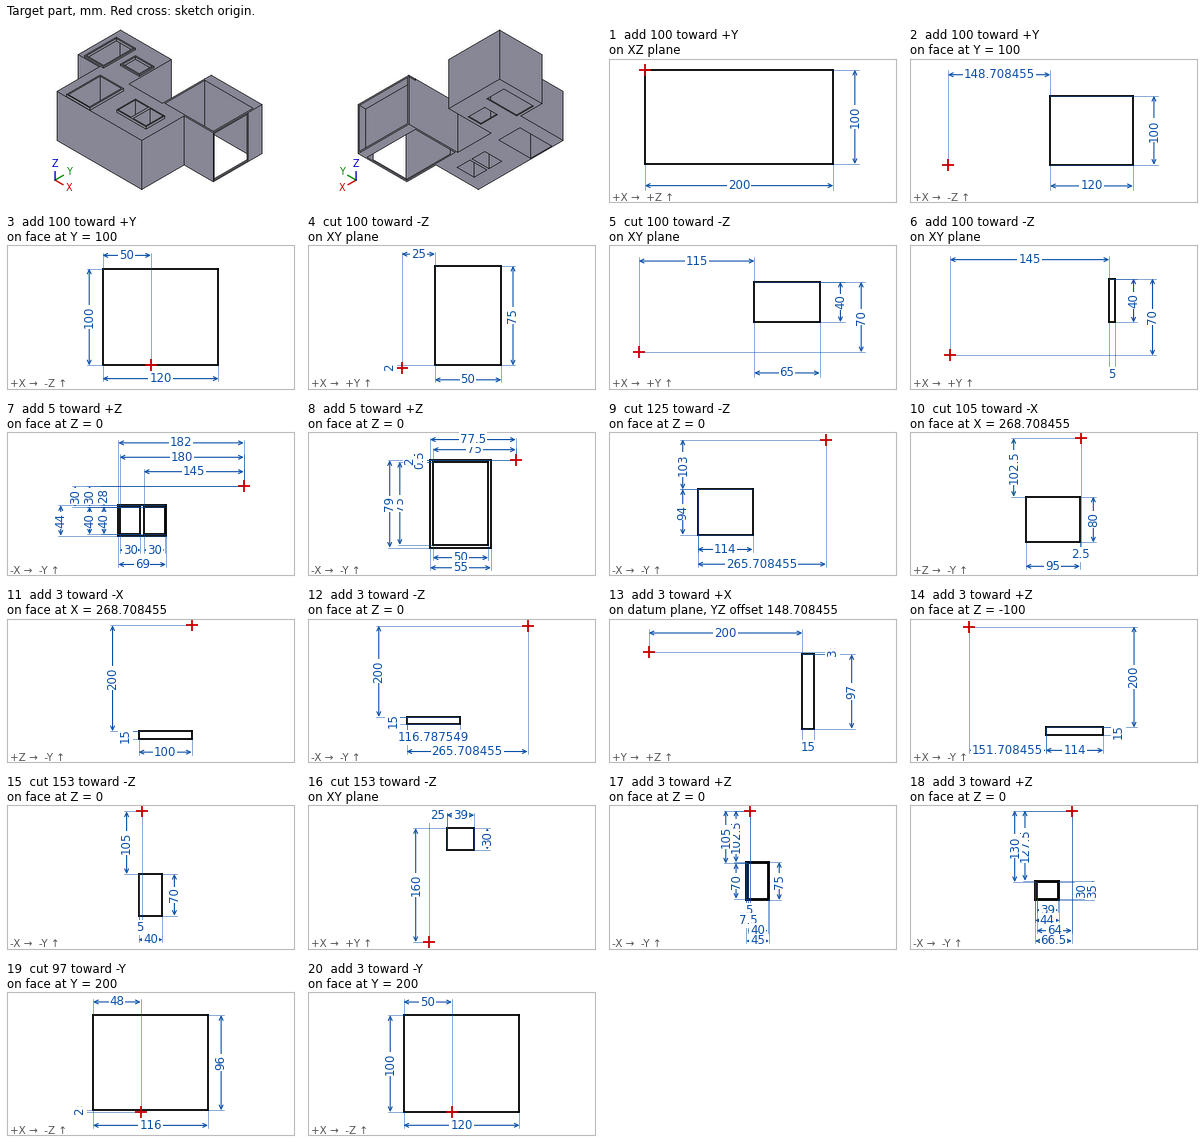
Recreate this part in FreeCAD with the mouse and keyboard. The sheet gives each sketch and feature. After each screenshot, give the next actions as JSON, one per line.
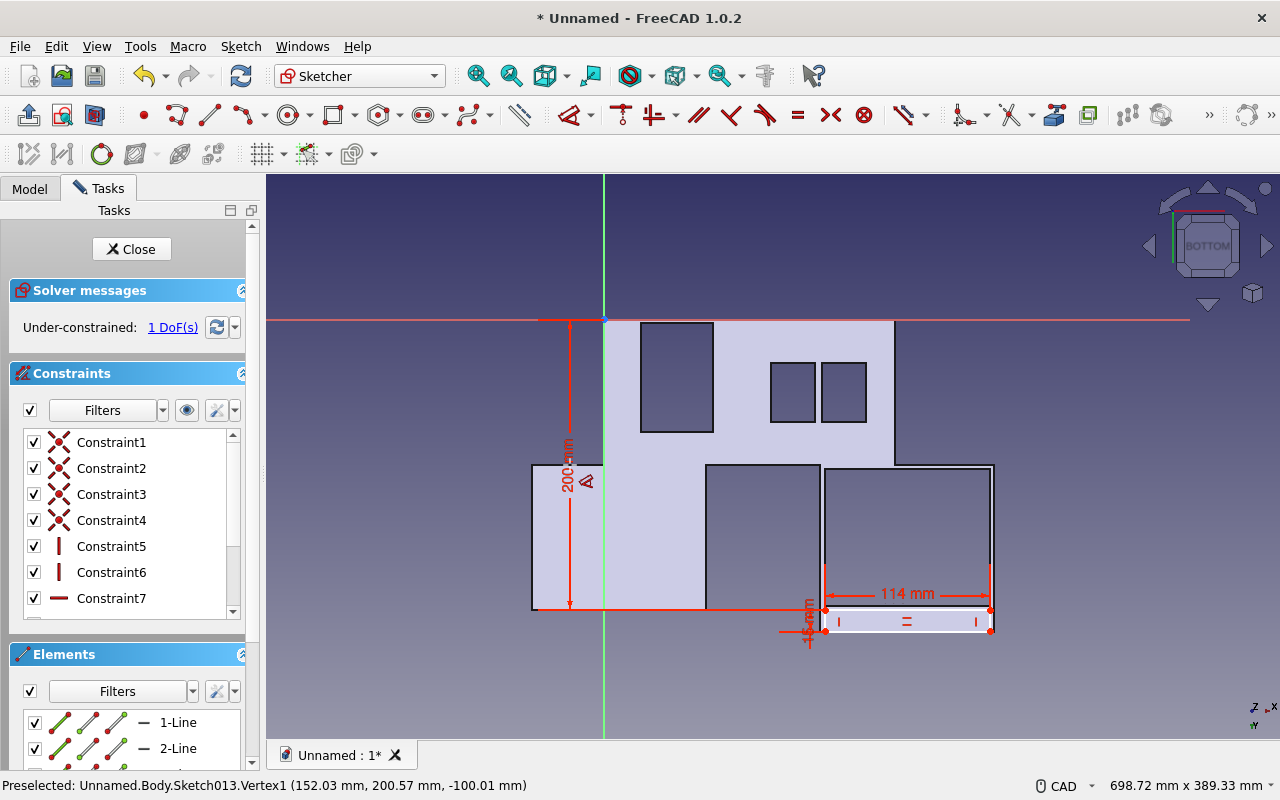
{"action": "left_click", "coordinate": [825, 610]}
{"action": "left_click", "coordinate": [715, 286]}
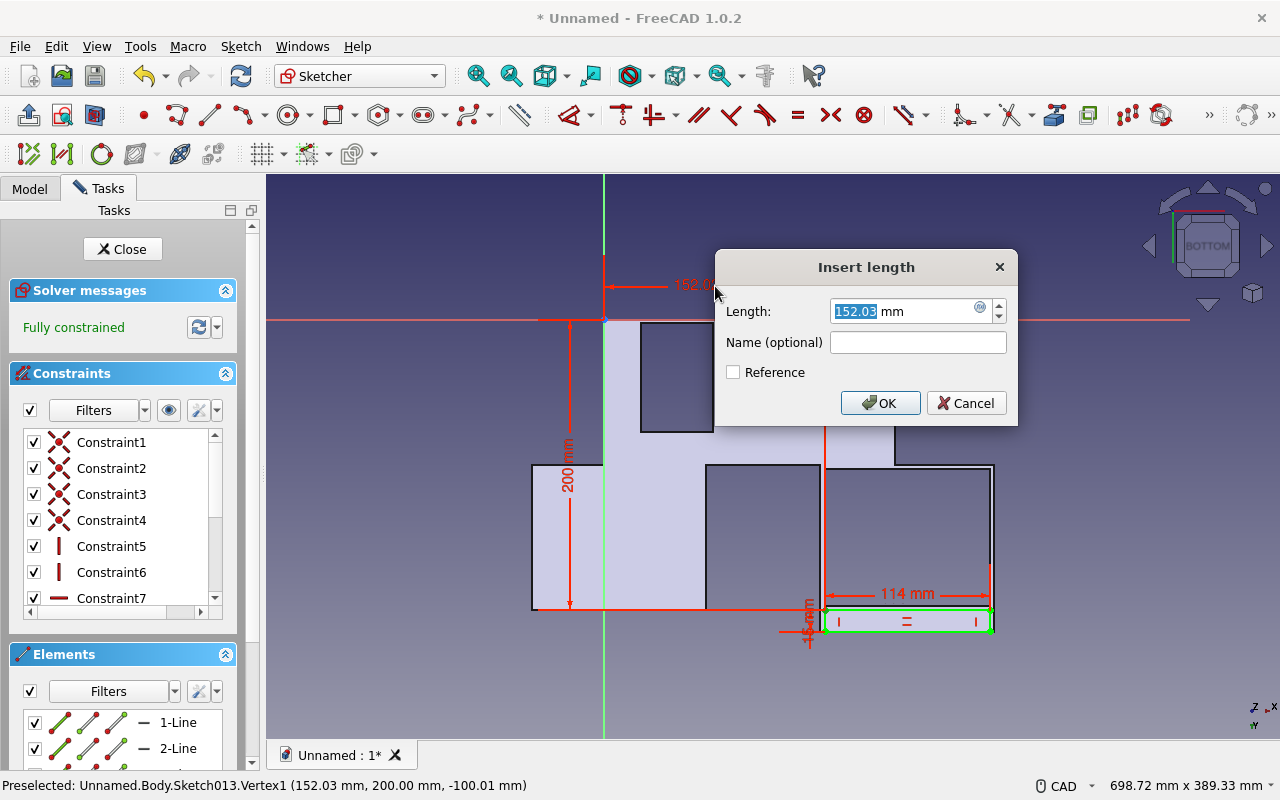
{"action": "type", "text": "151.708455"}
{"action": "key", "text": "Return"}
{"action": "key", "text": "Escape"}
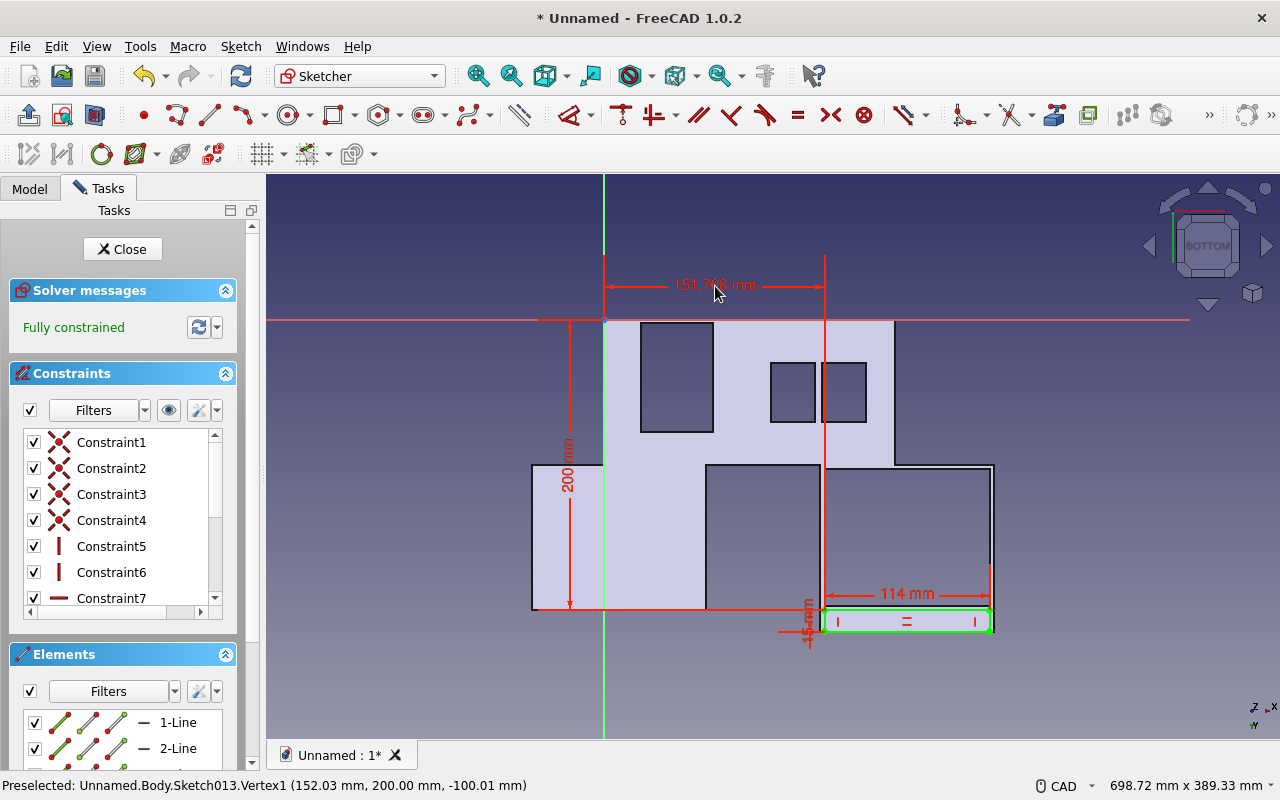
{"action": "left_click", "coordinate": [123, 249]}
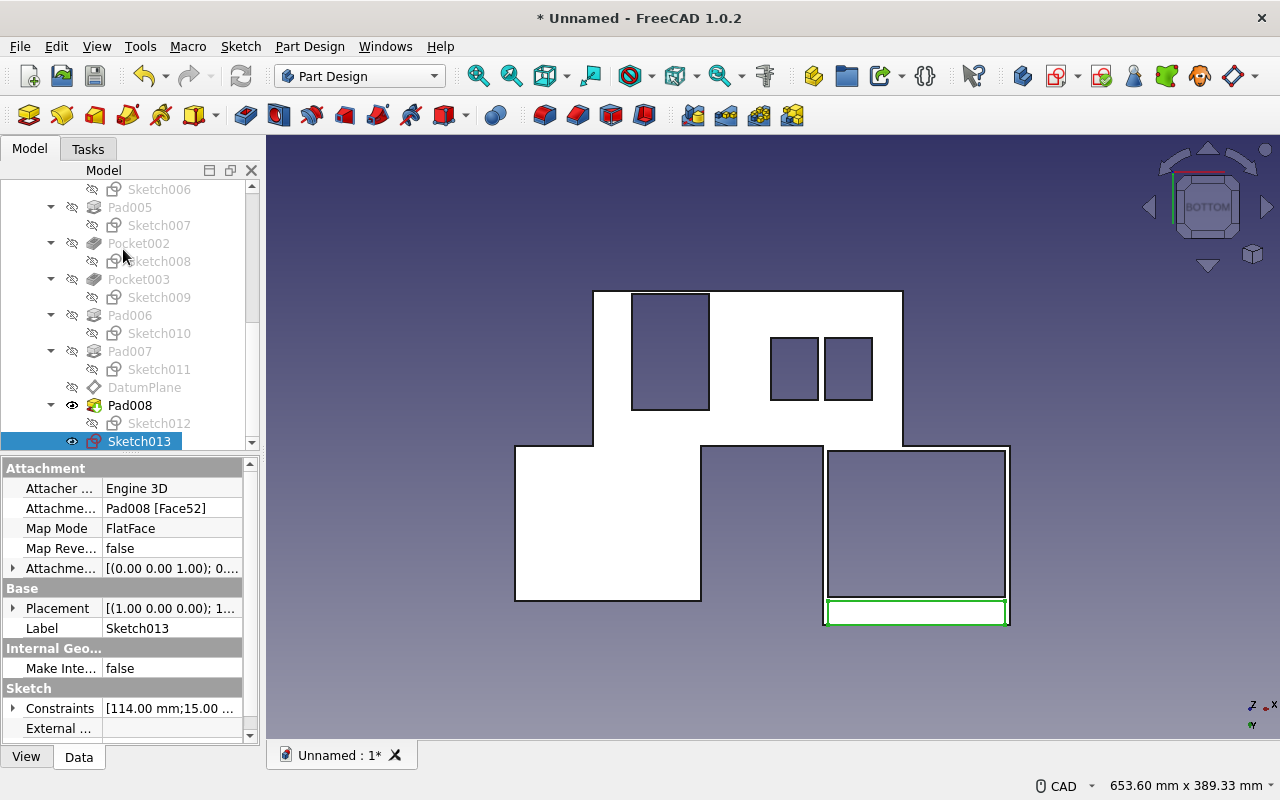
{"action": "left_click", "coordinate": [29, 116]}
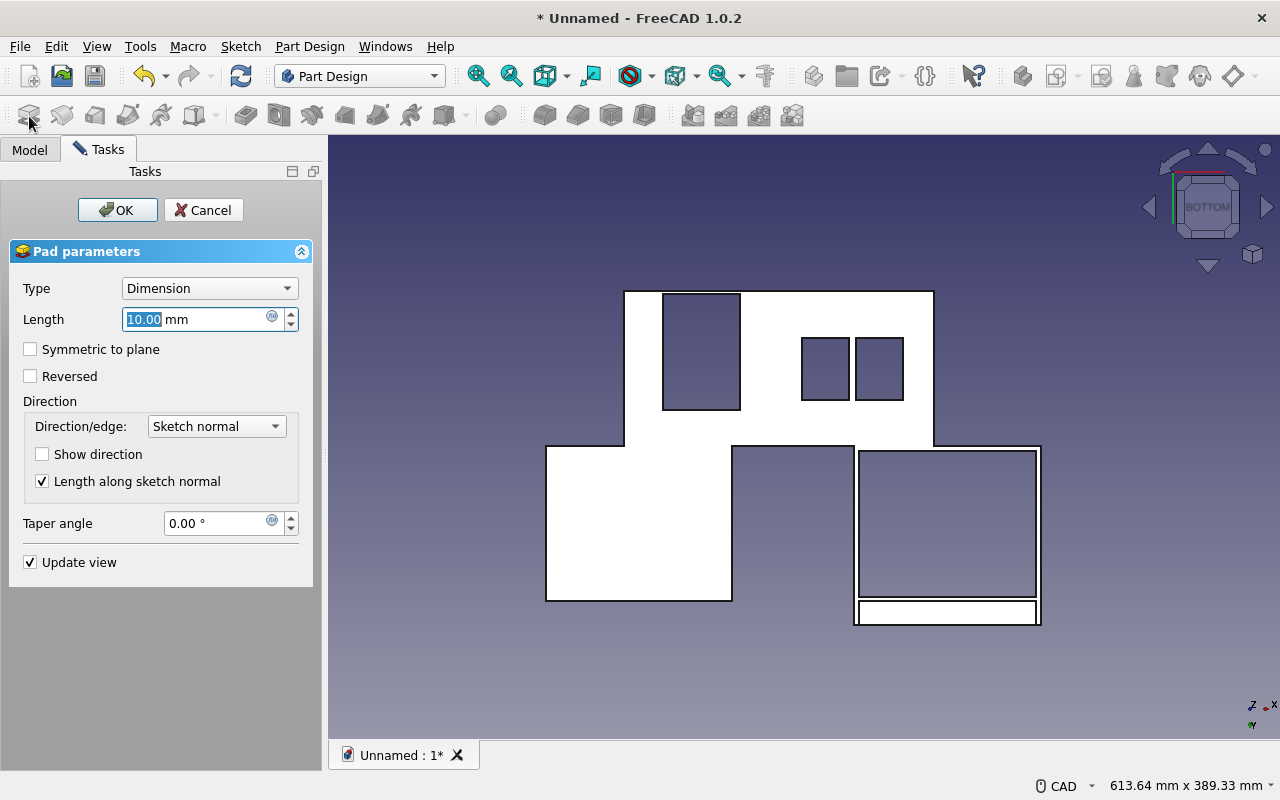
{"action": "type", "text": "3"}
{"action": "key", "text": "Tab"}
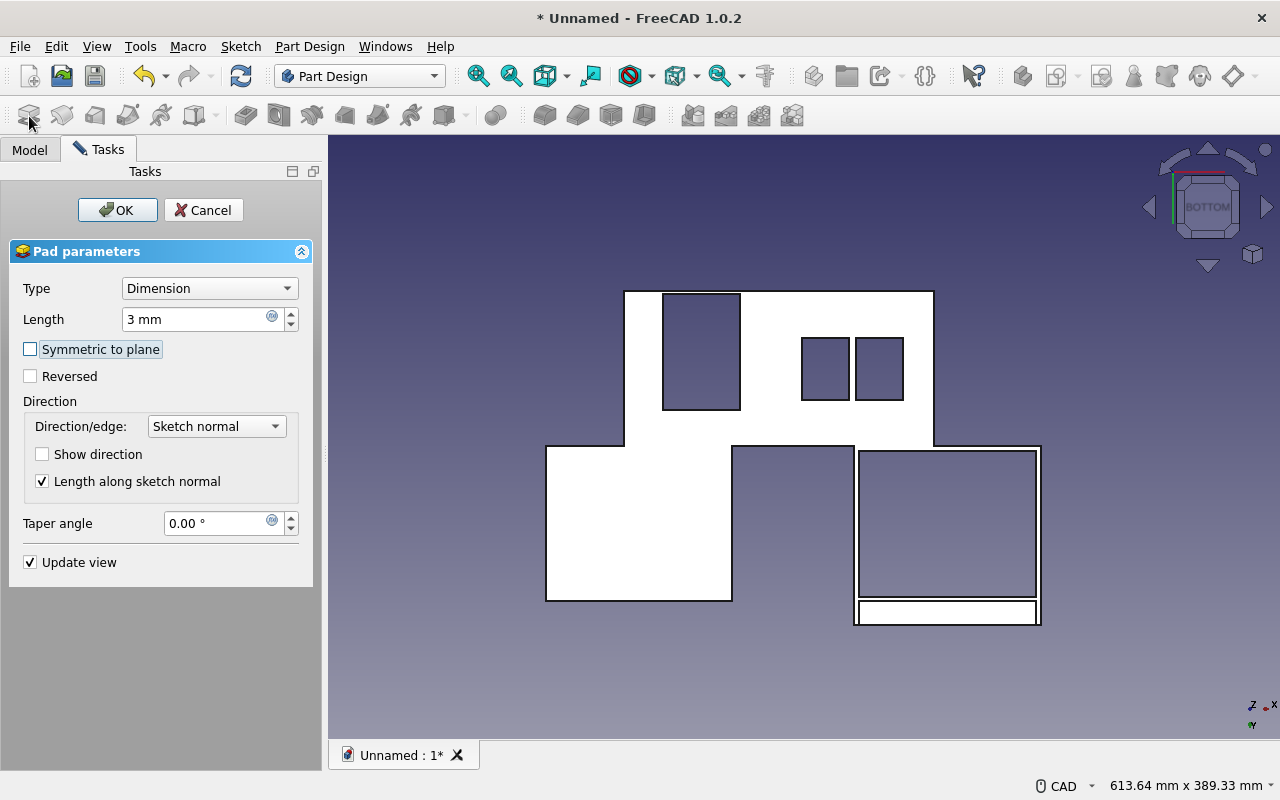
{"action": "left_click", "coordinate": [31, 376]}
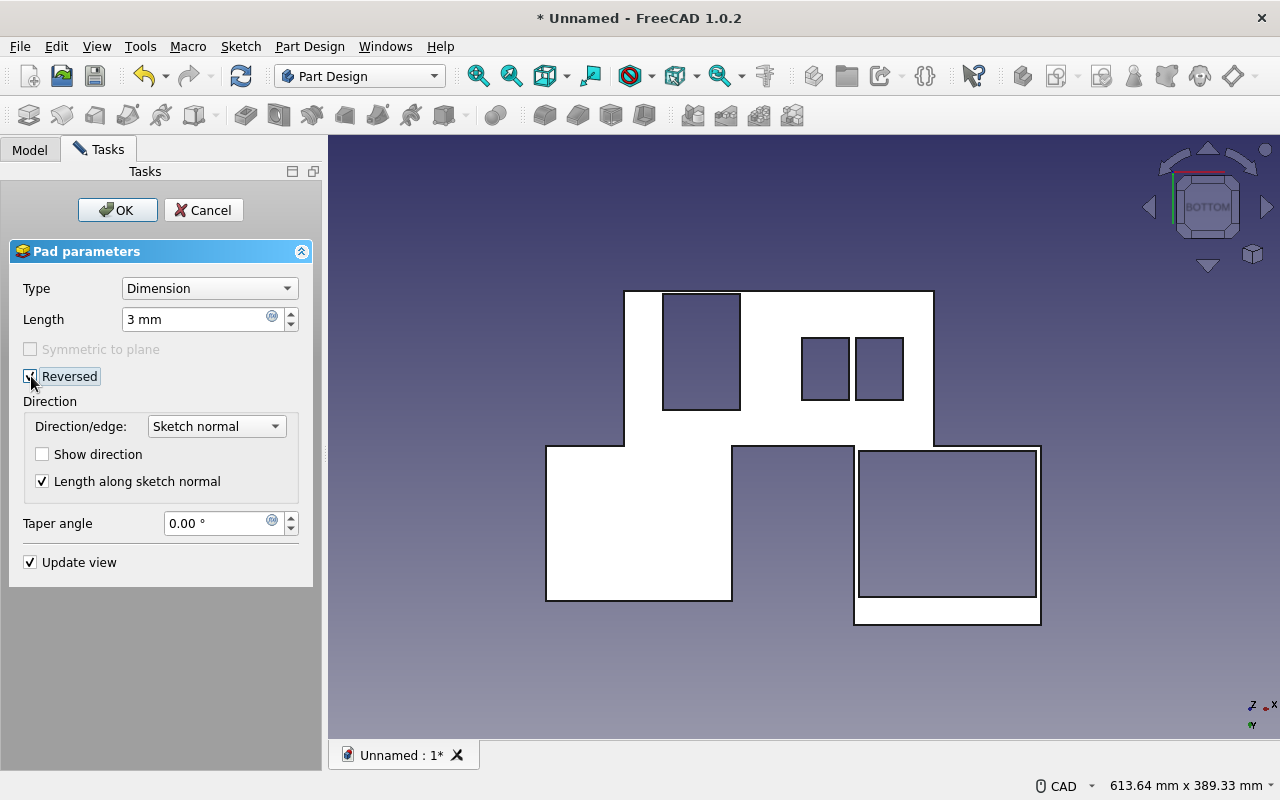
{"action": "left_click", "coordinate": [118, 210]}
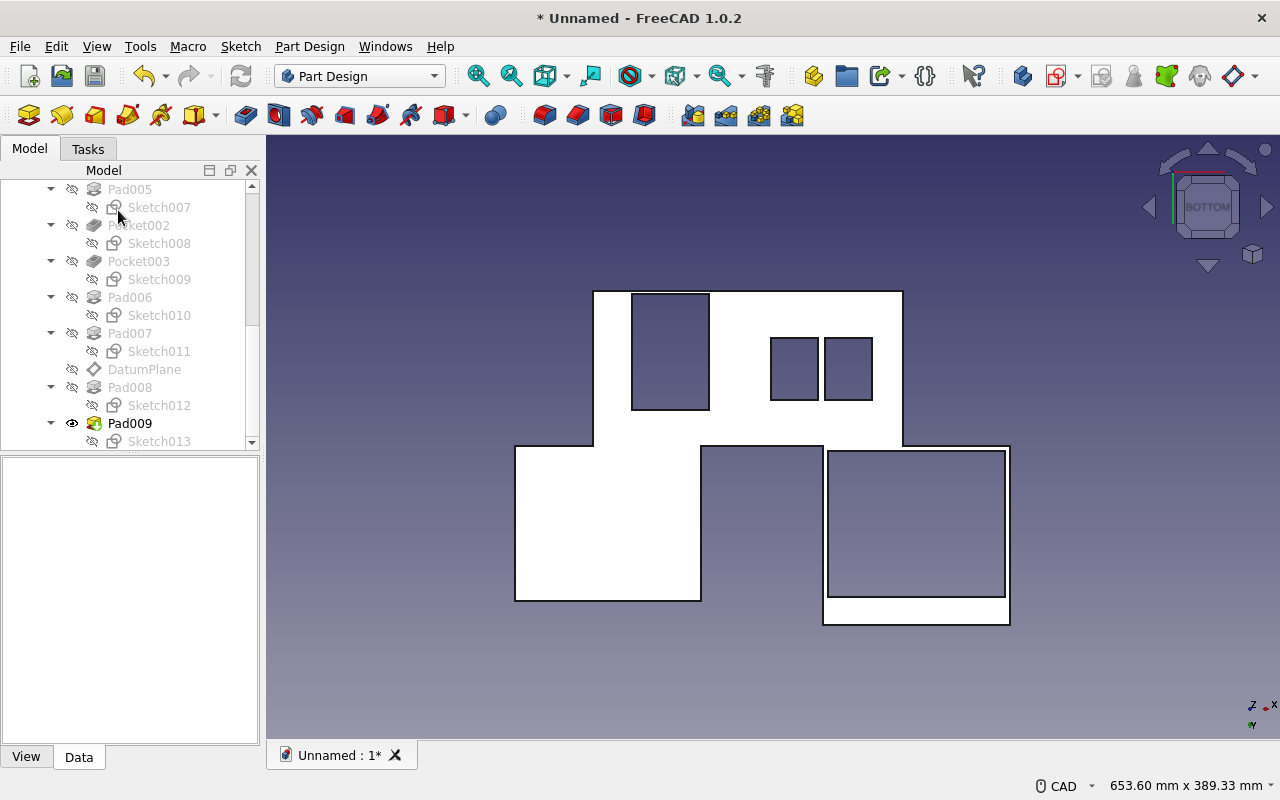
{"action": "key", "text": "0"}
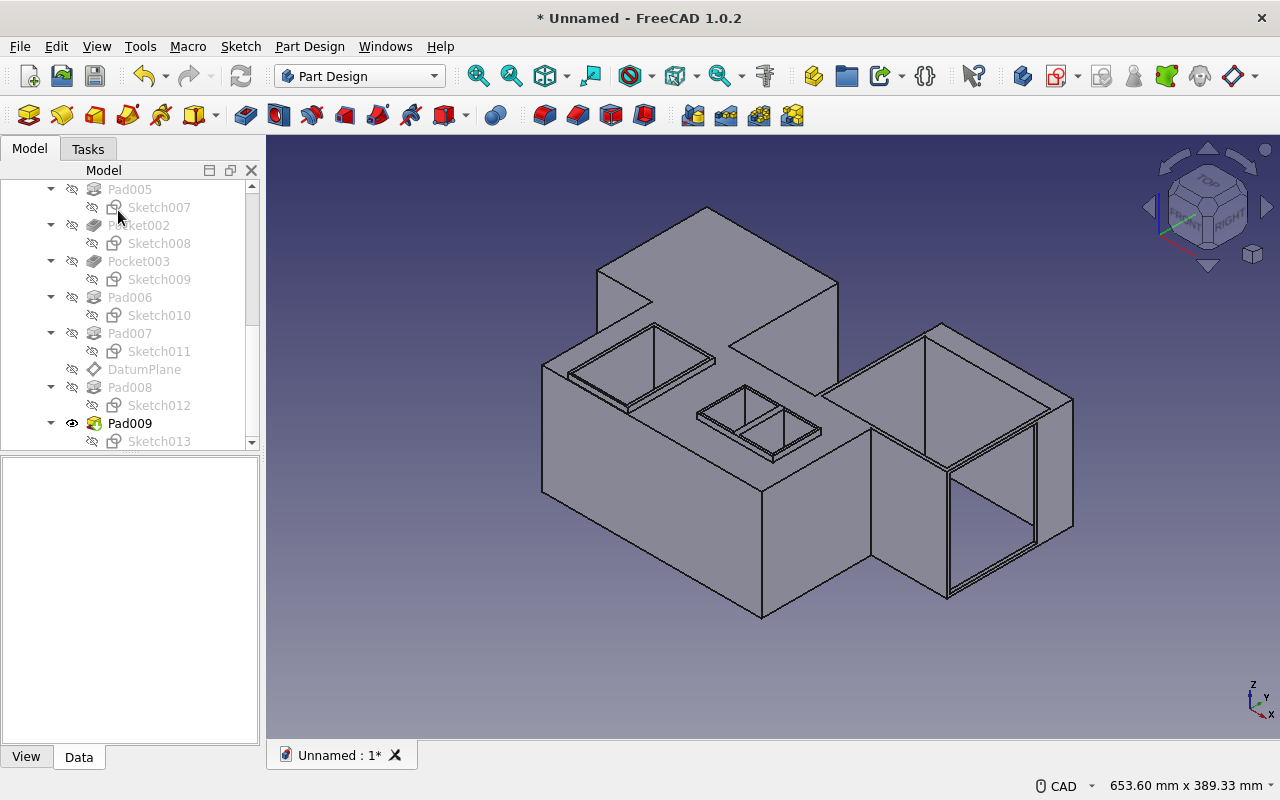
{"action": "left_click", "coordinate": [714, 288]}